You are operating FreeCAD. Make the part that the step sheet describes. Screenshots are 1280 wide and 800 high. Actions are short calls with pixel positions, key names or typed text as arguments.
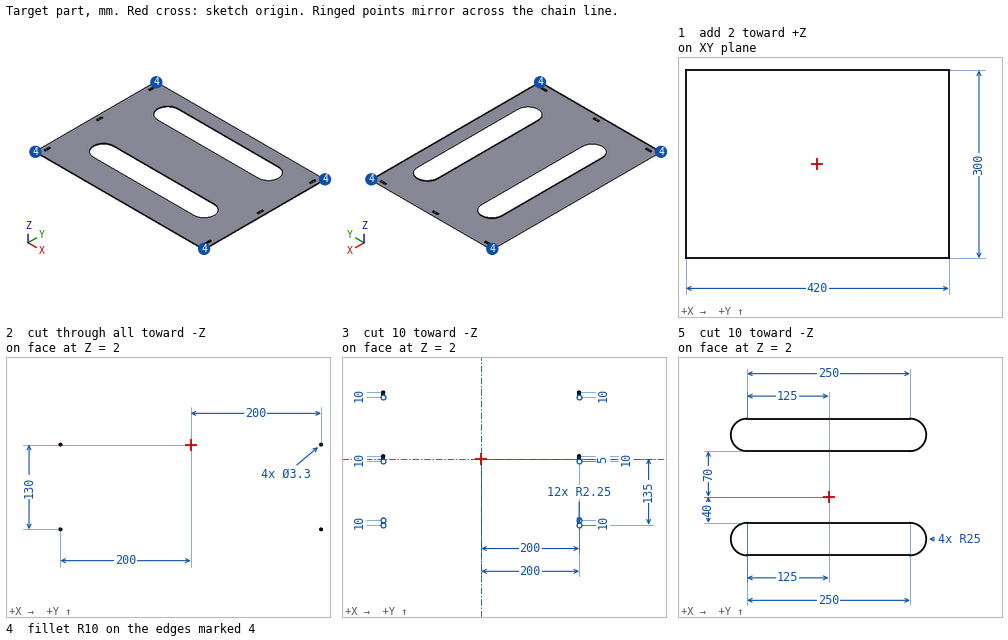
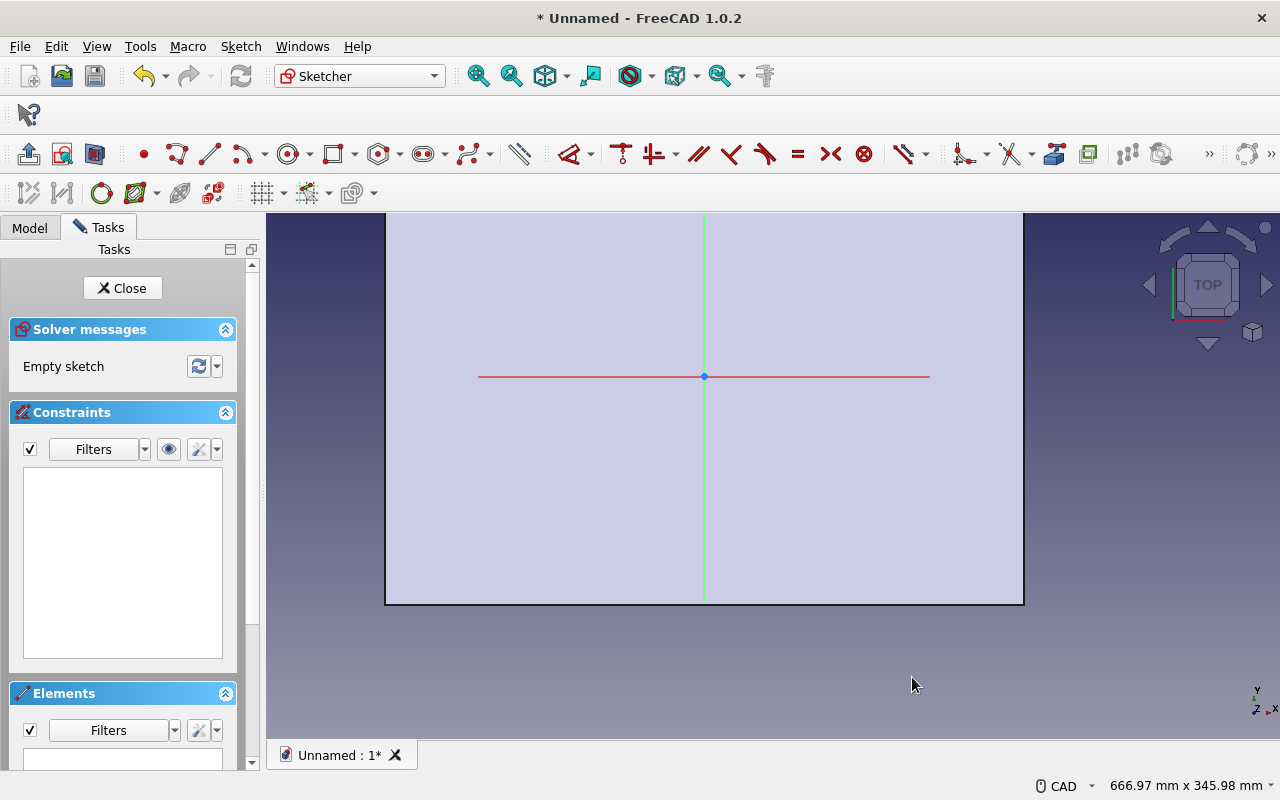
click(288, 154)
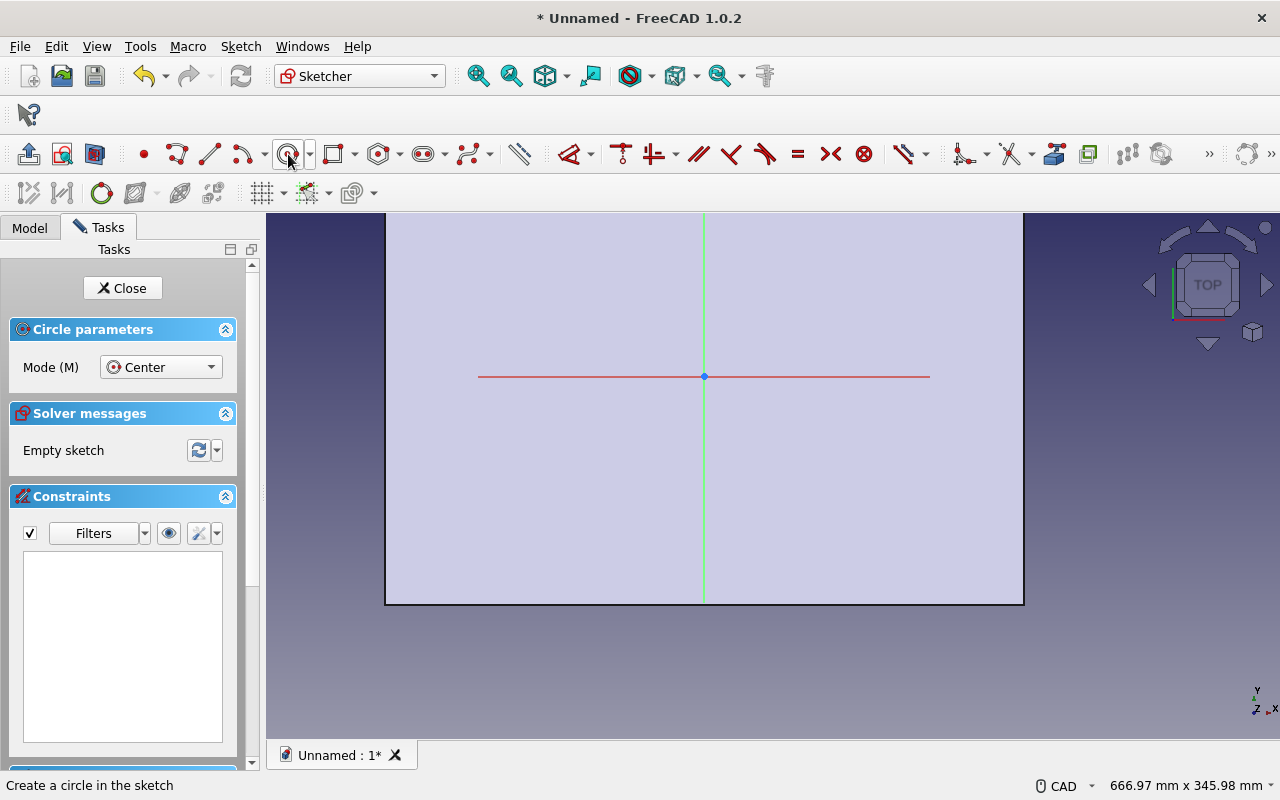
scroll(1008, 377, up, 12)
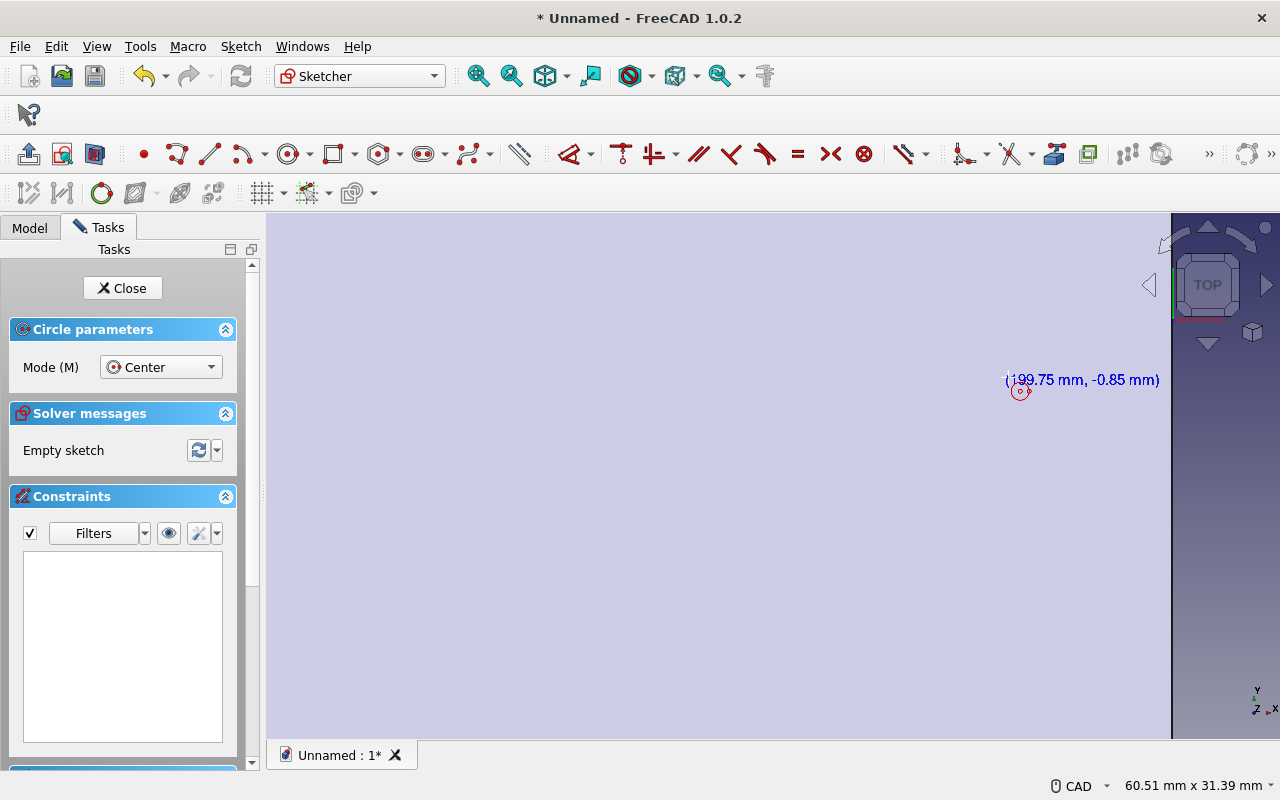
scroll(1009, 378, down, 12)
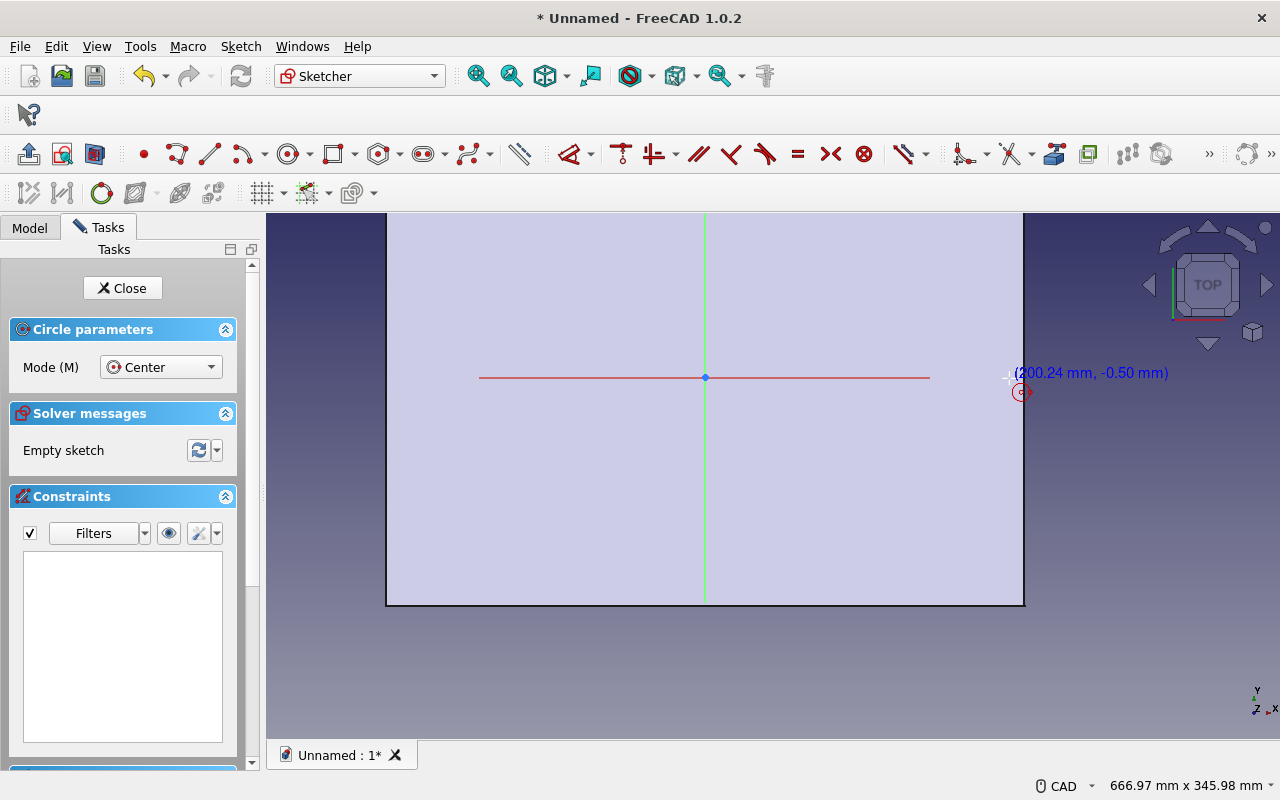
click(1009, 378)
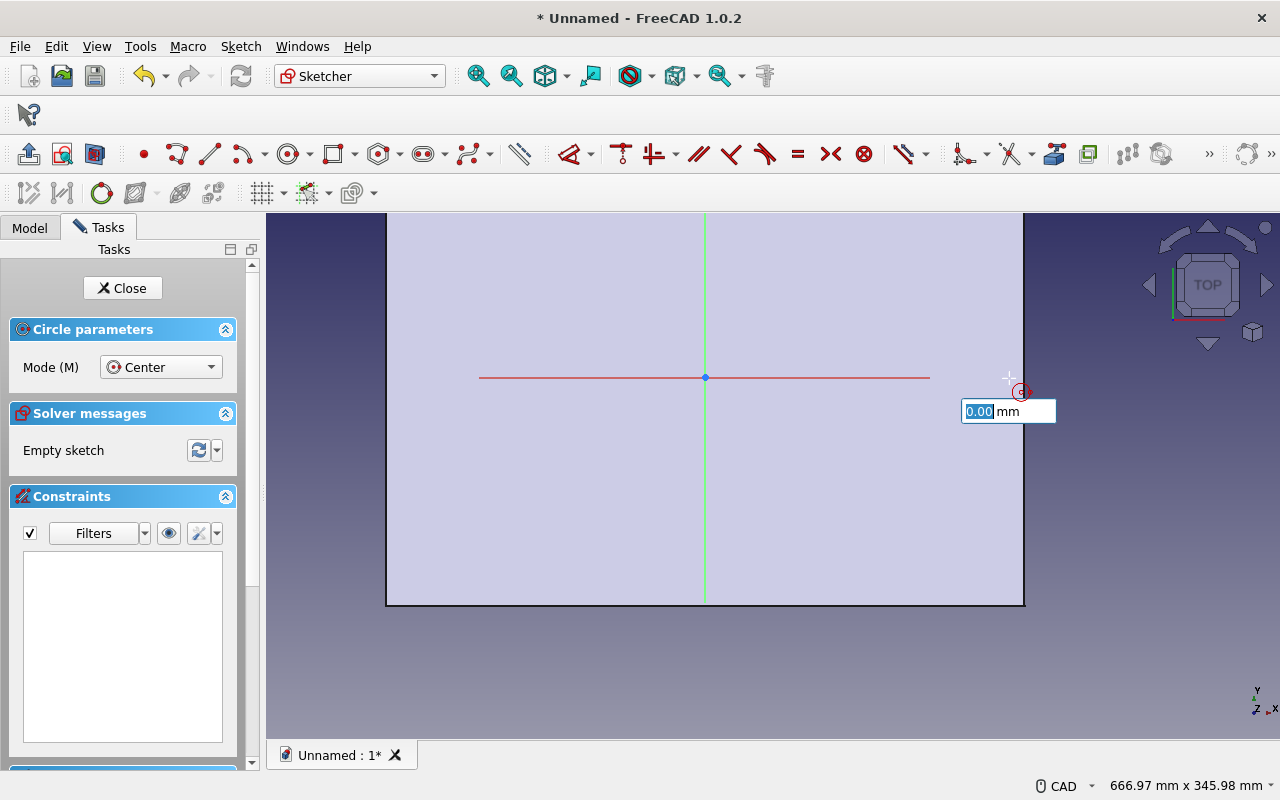
scroll(1008, 380, up, 10)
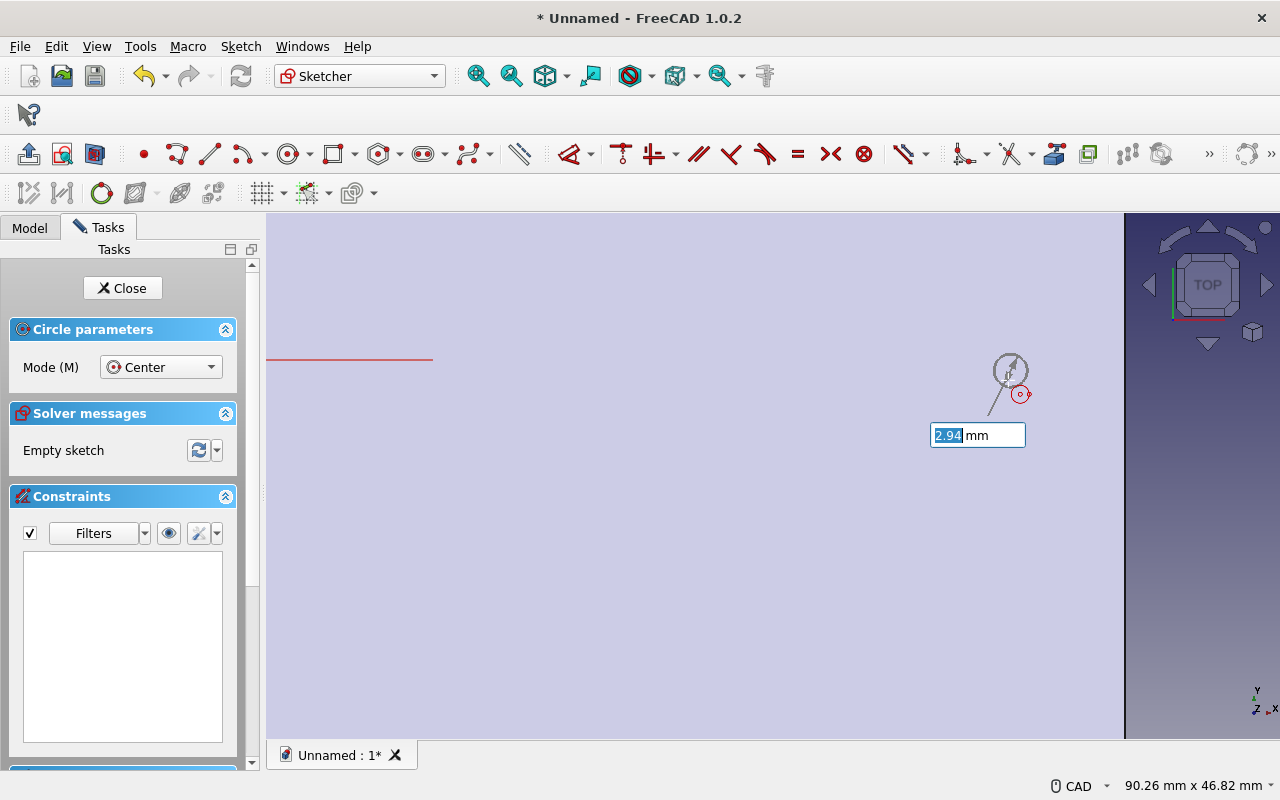
click(1007, 378)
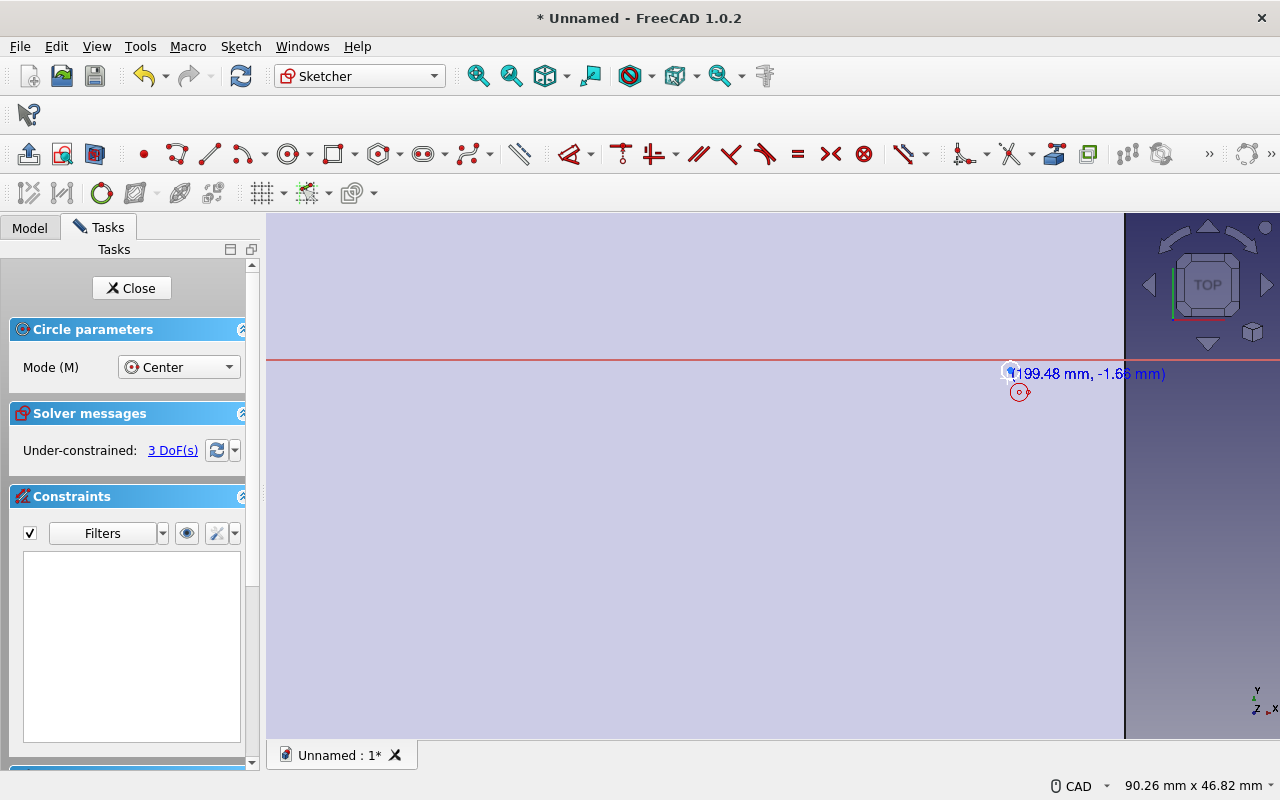
scroll(1008, 380, down, 10)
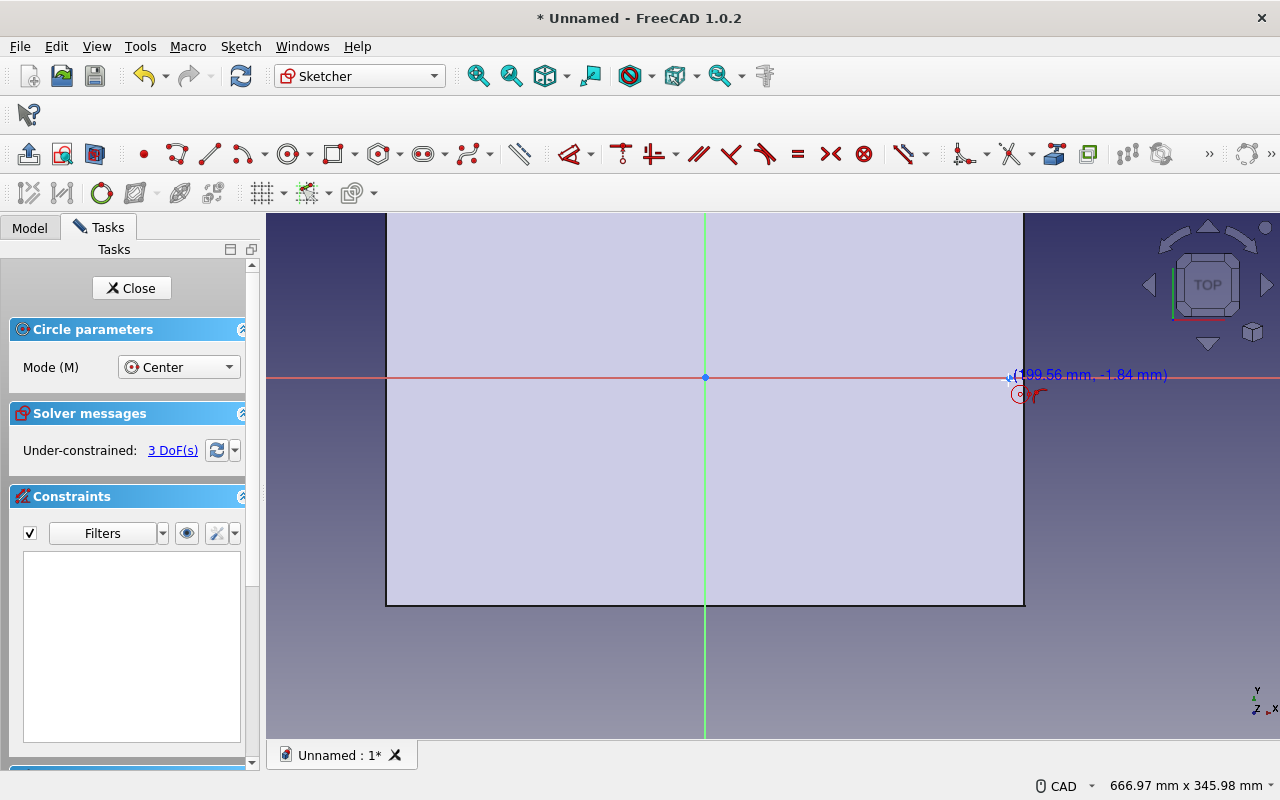
scroll(401, 575, up, 12)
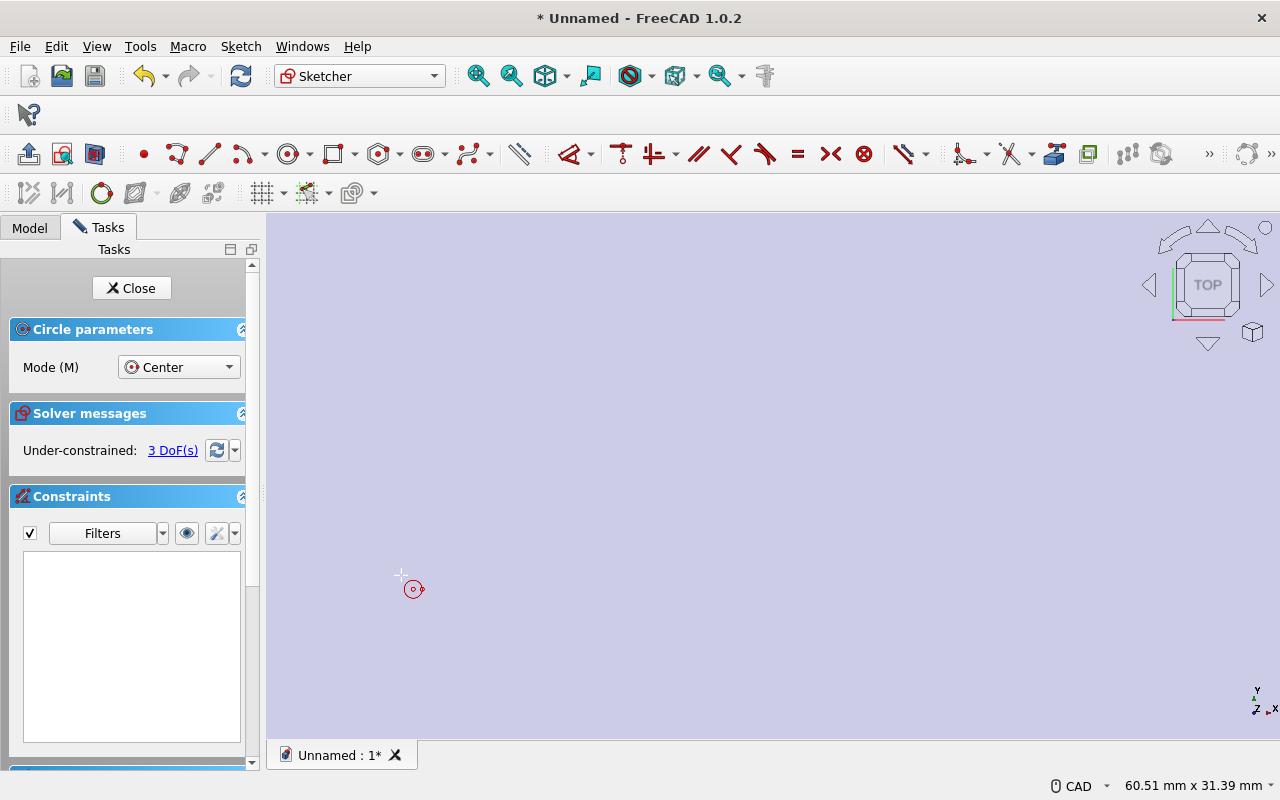
scroll(400, 575, down, 12)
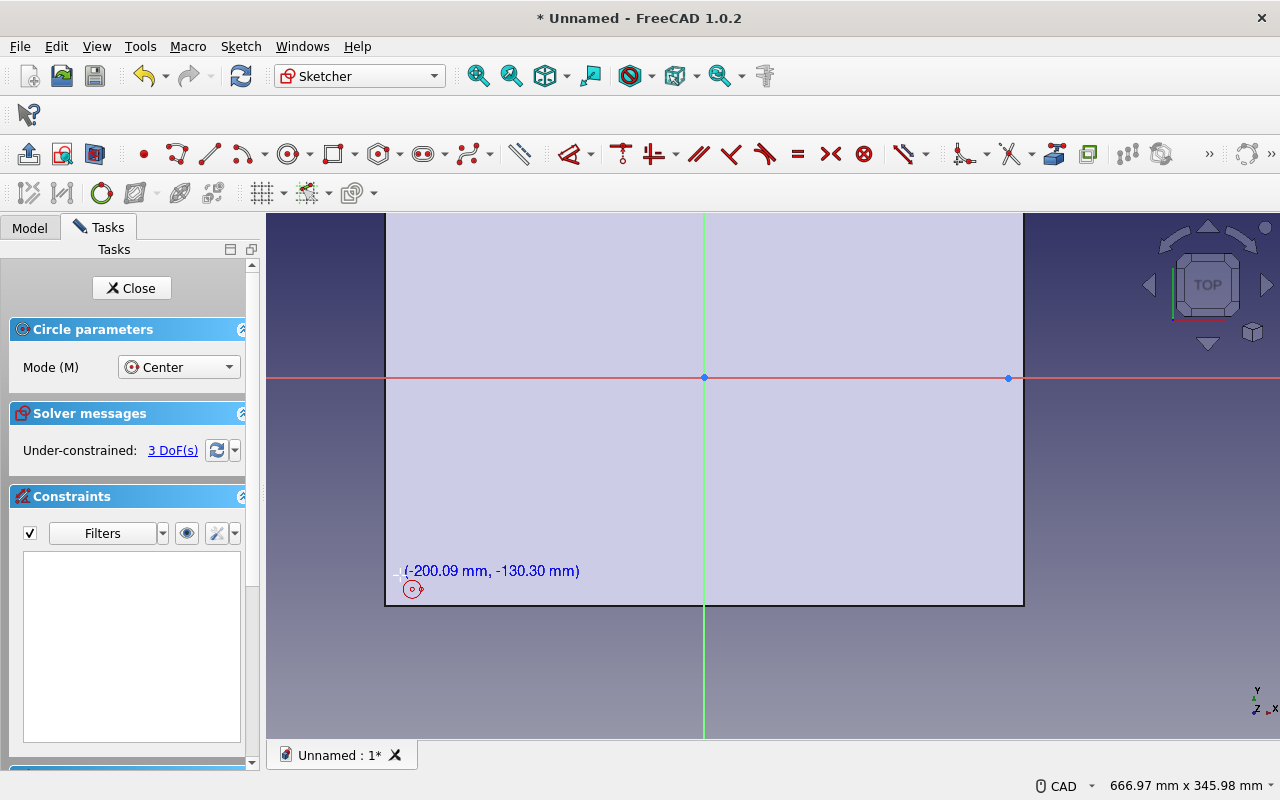
click(400, 575)